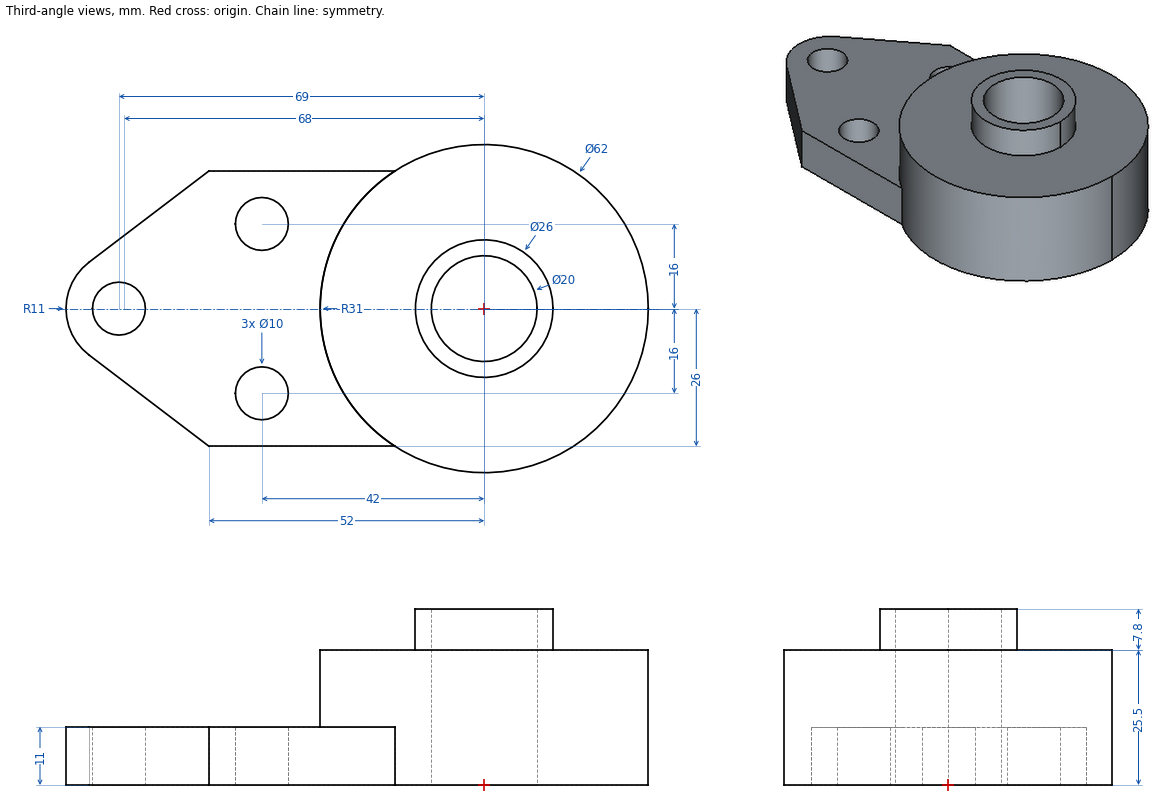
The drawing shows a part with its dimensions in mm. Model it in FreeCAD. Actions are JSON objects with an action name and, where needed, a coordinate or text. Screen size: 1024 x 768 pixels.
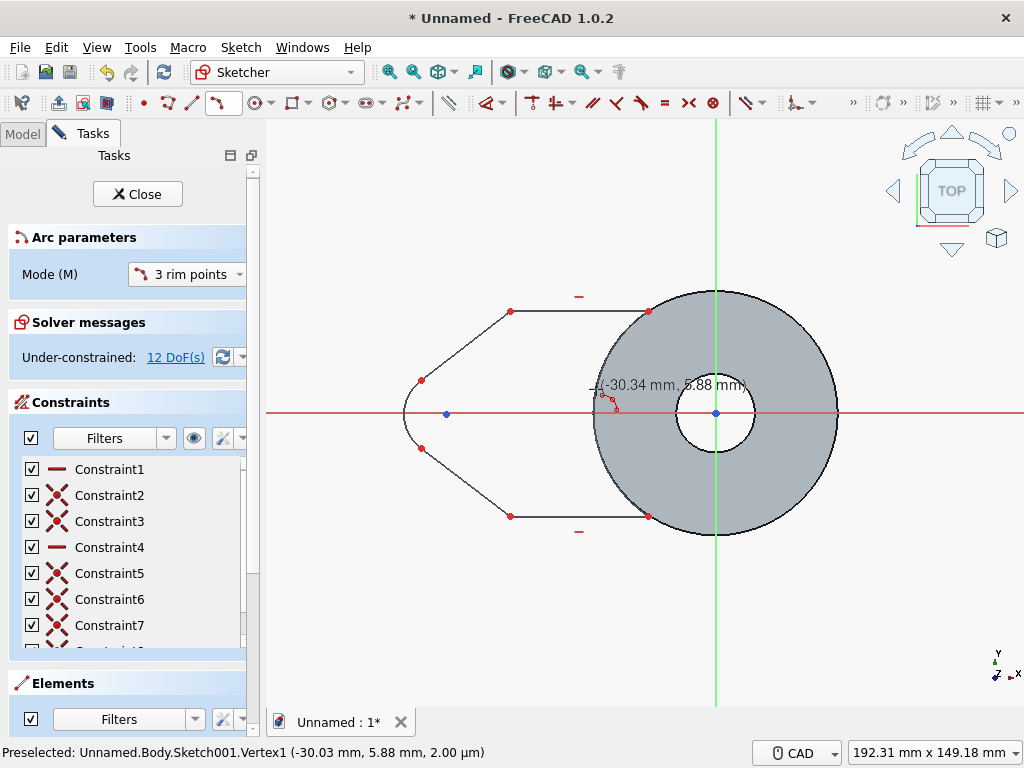
{"action": "left_click", "coordinate": [256, 104]}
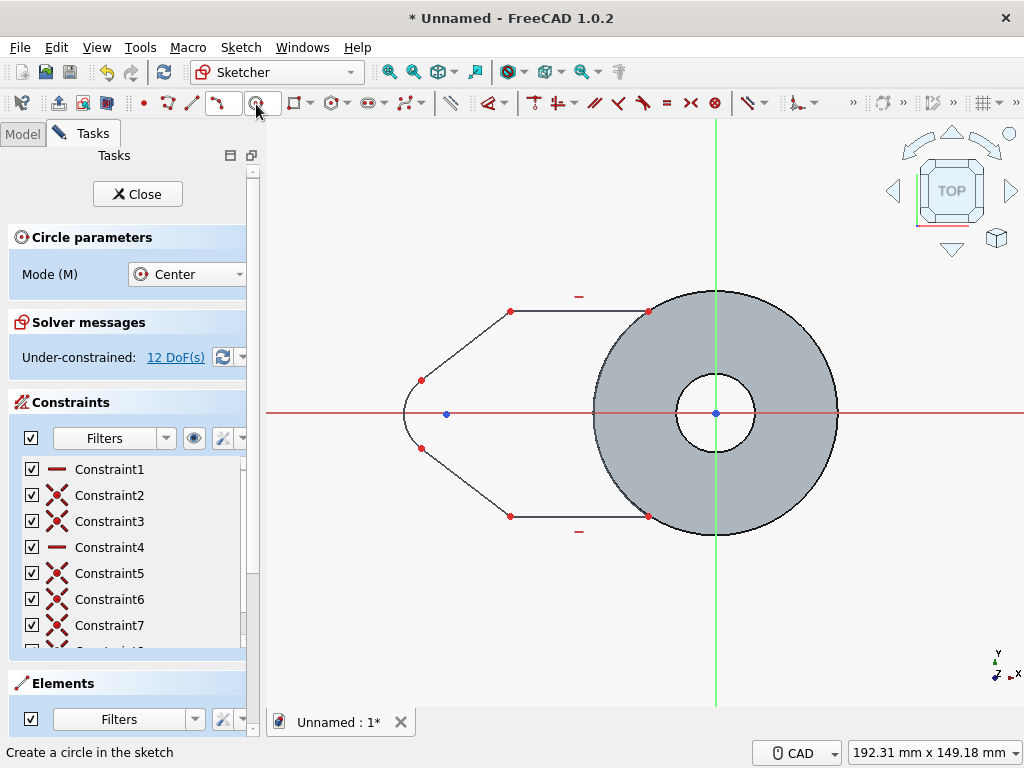
{"action": "left_click", "coordinate": [550, 476]}
{"action": "mouse_move", "coordinate": [564, 462]}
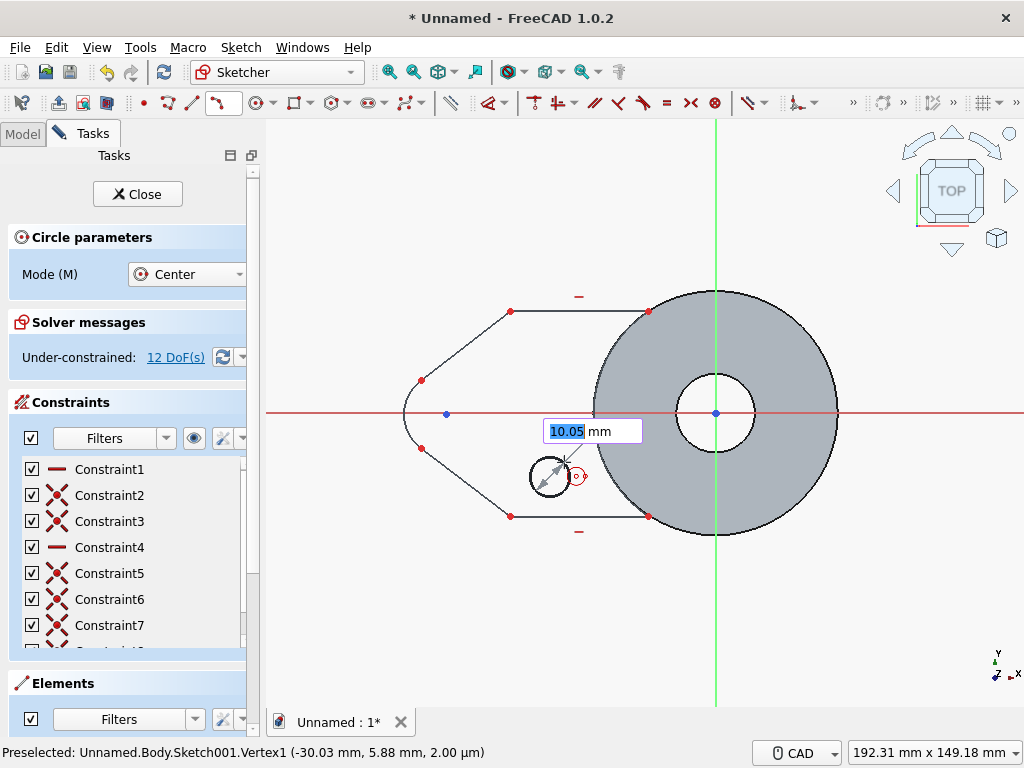
{"action": "type", "text": "10"}
{"action": "key", "text": "Return"}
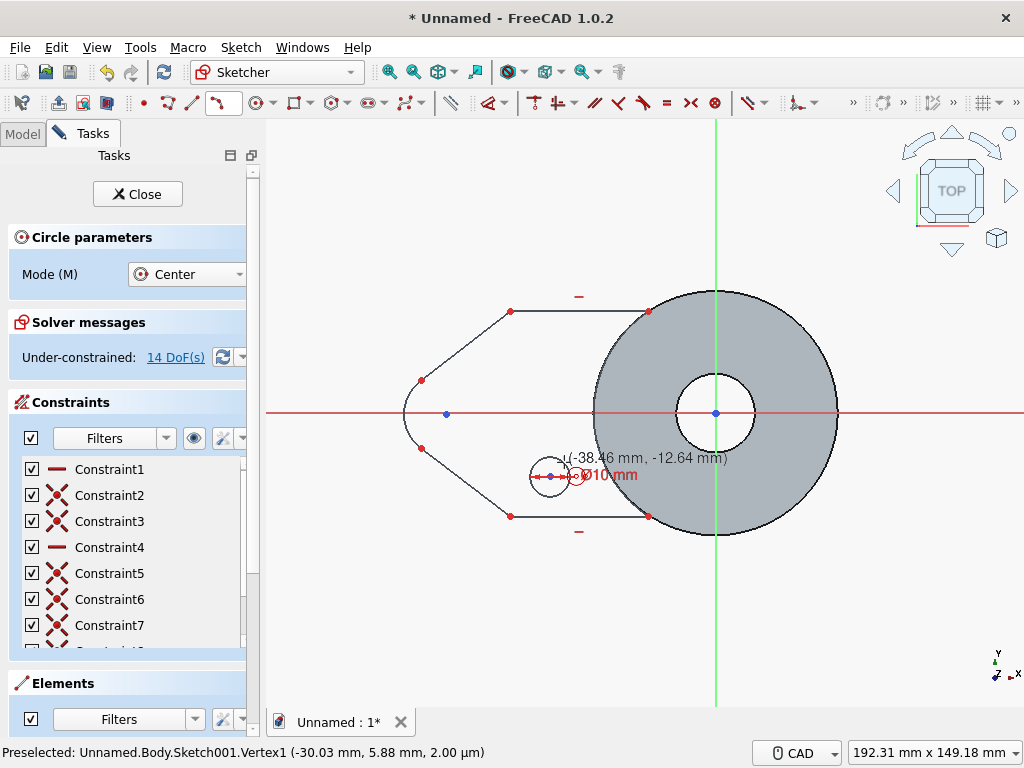
{"action": "scroll", "coordinate": [444, 413], "scroll_direction": "up", "scroll_amount": 7}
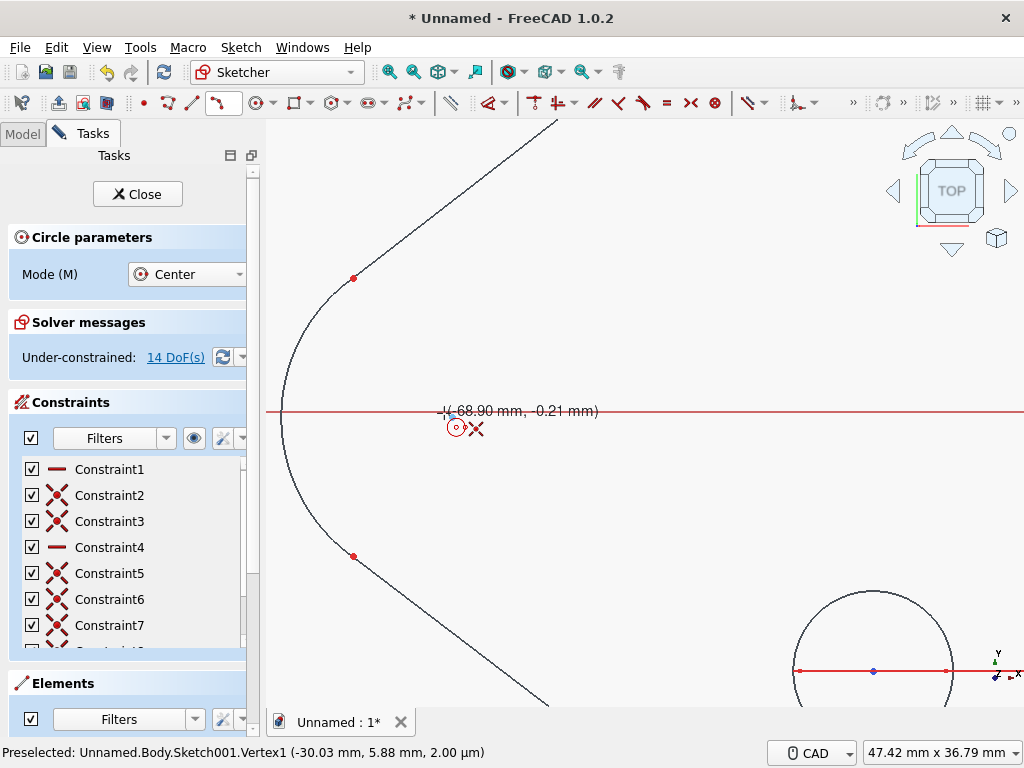
{"action": "left_click", "coordinate": [442, 412]}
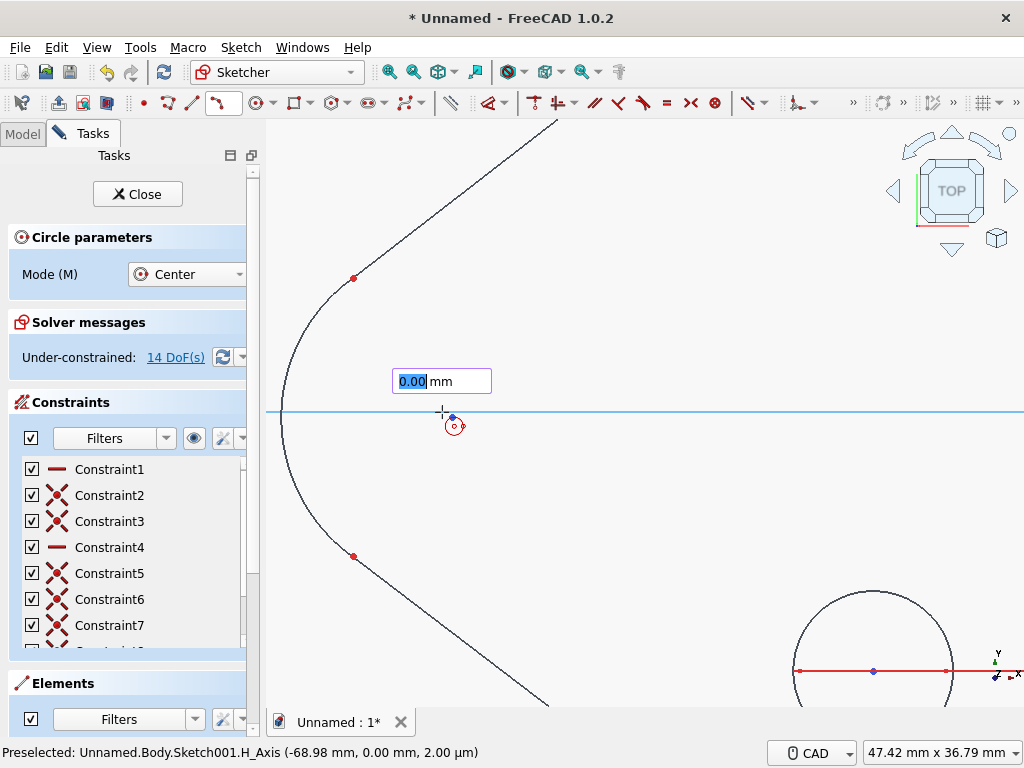
{"action": "scroll", "coordinate": [431, 413], "scroll_direction": "down", "scroll_amount": 6}
{"action": "mouse_move", "coordinate": [451, 396]}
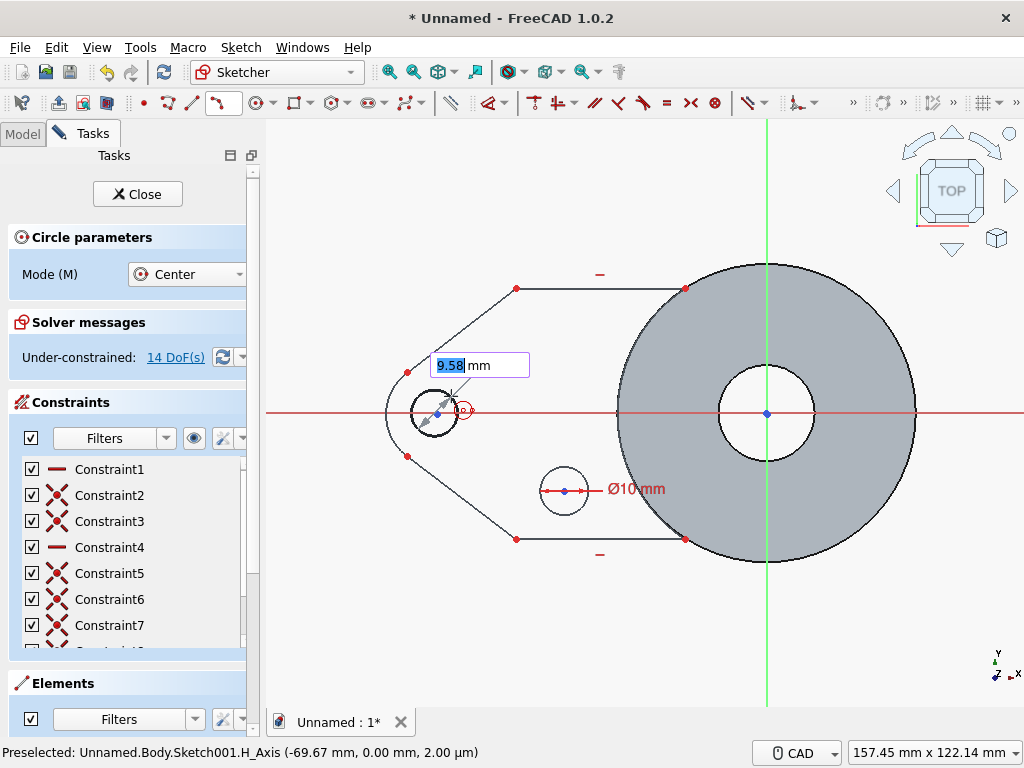
{"action": "type", "text": "10"}
{"action": "key", "text": "Return"}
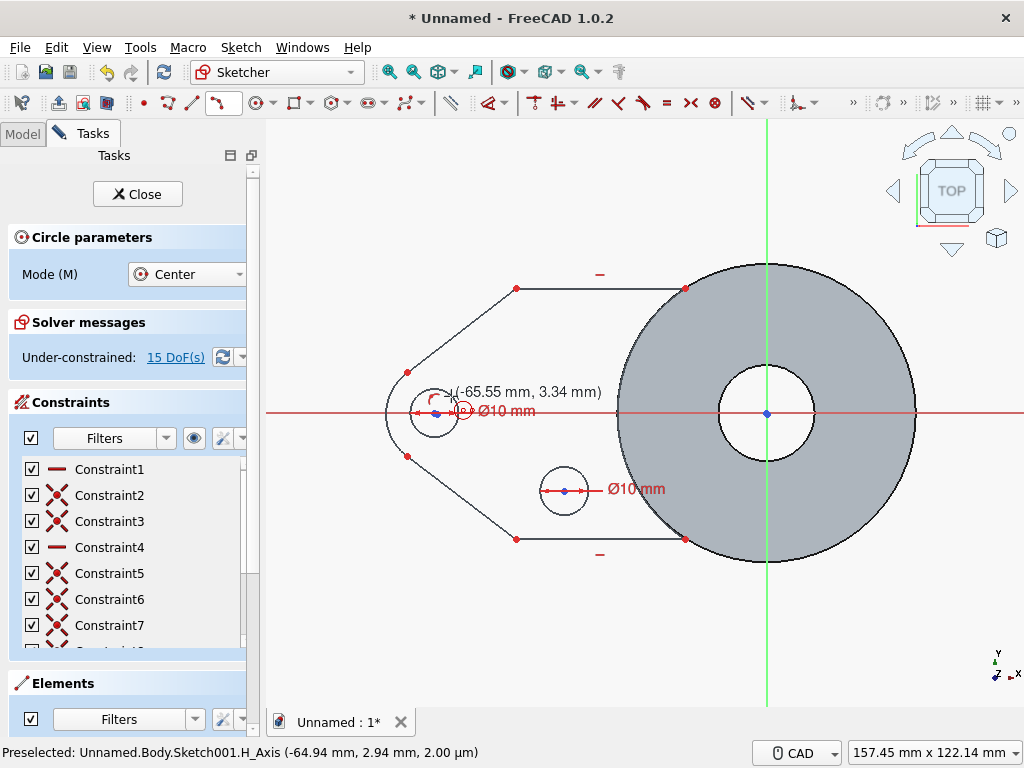
{"action": "left_click", "coordinate": [564, 336]}
{"action": "mouse_move", "coordinate": [581, 319]}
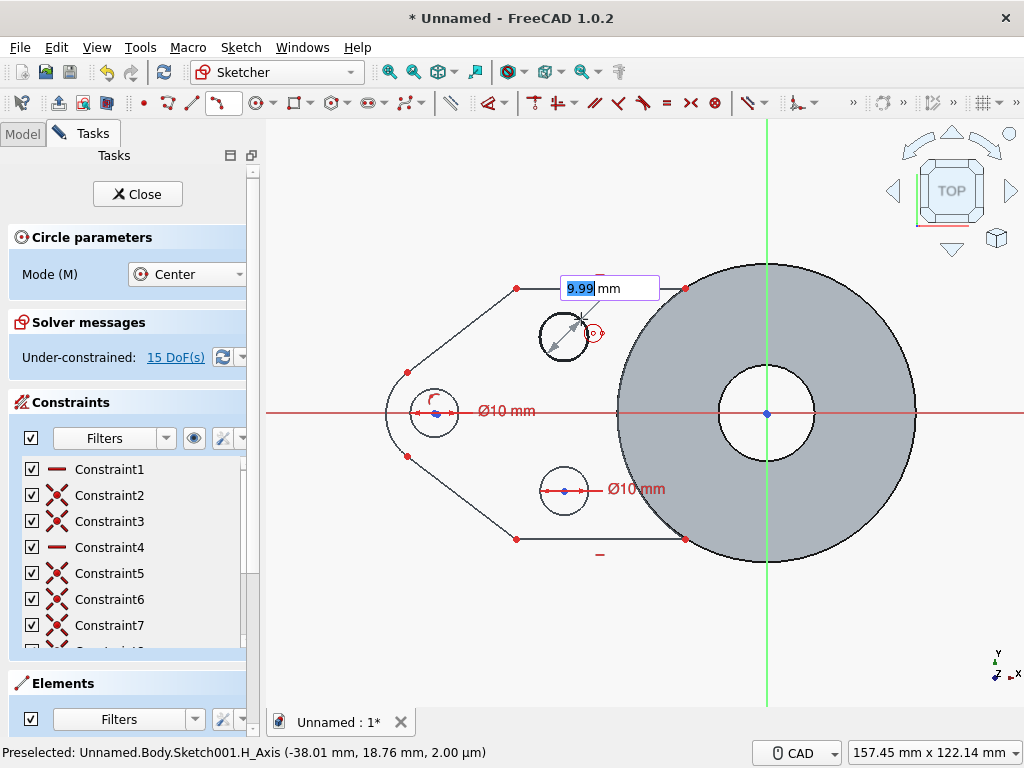
{"action": "type", "text": "10"}
{"action": "key", "text": "Return"}
{"action": "key", "text": "Escape"}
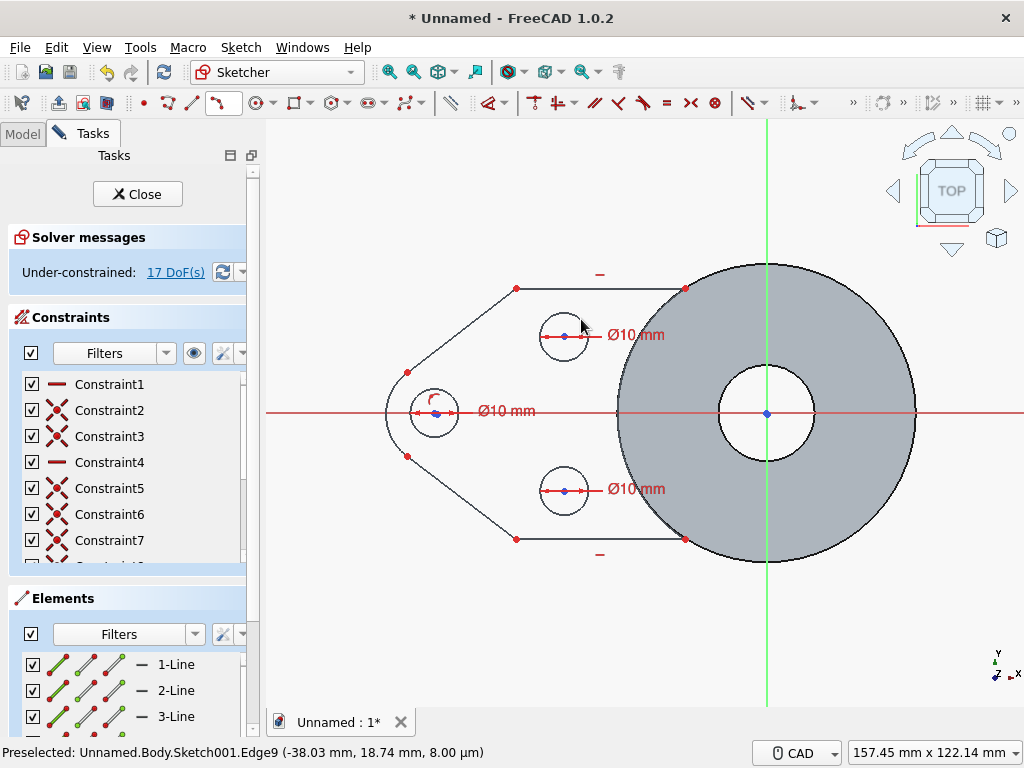
{"action": "left_click", "coordinate": [484, 515]}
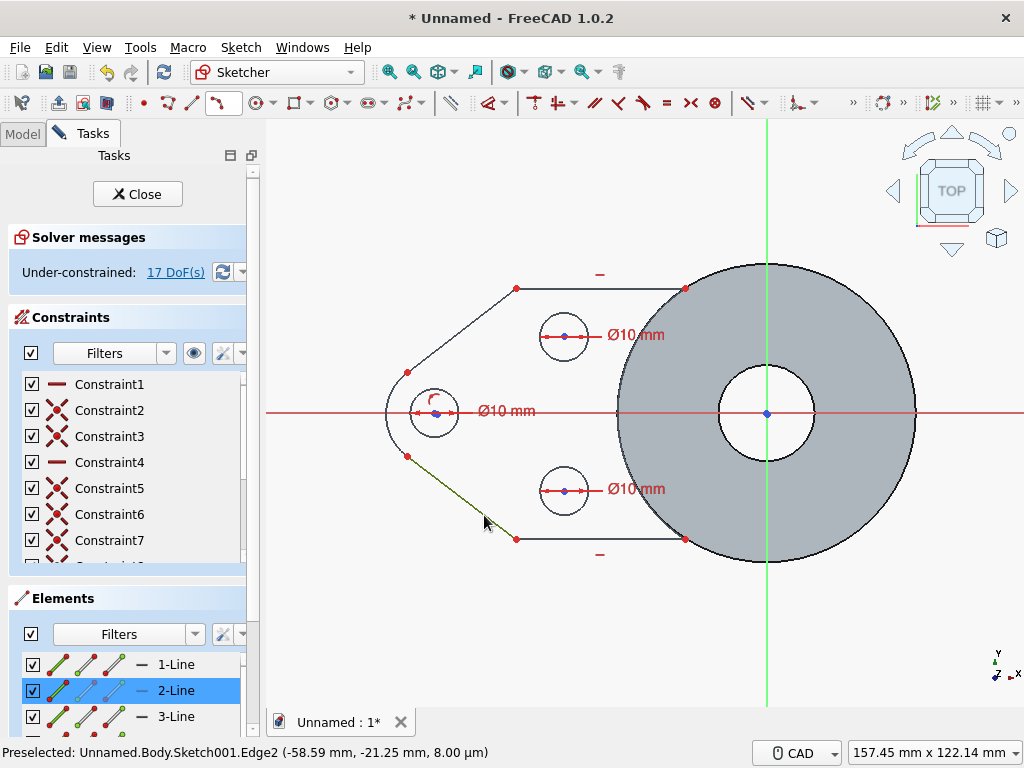
{"action": "left_click", "coordinate": [390, 396]}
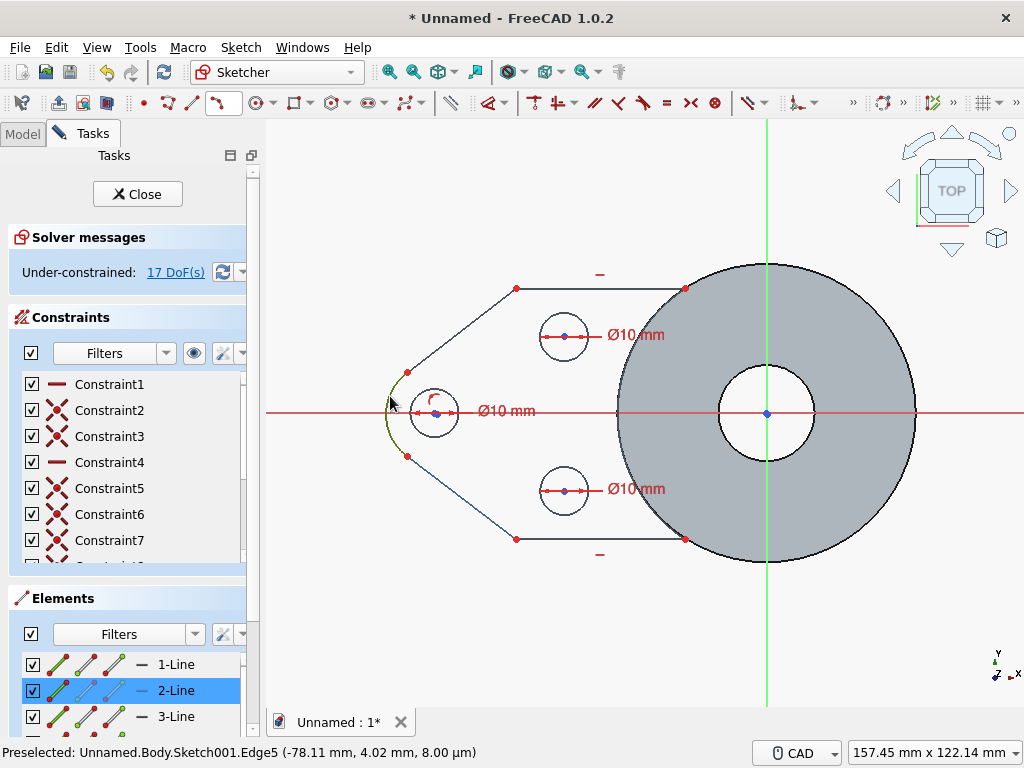
{"action": "left_click", "coordinate": [644, 104]}